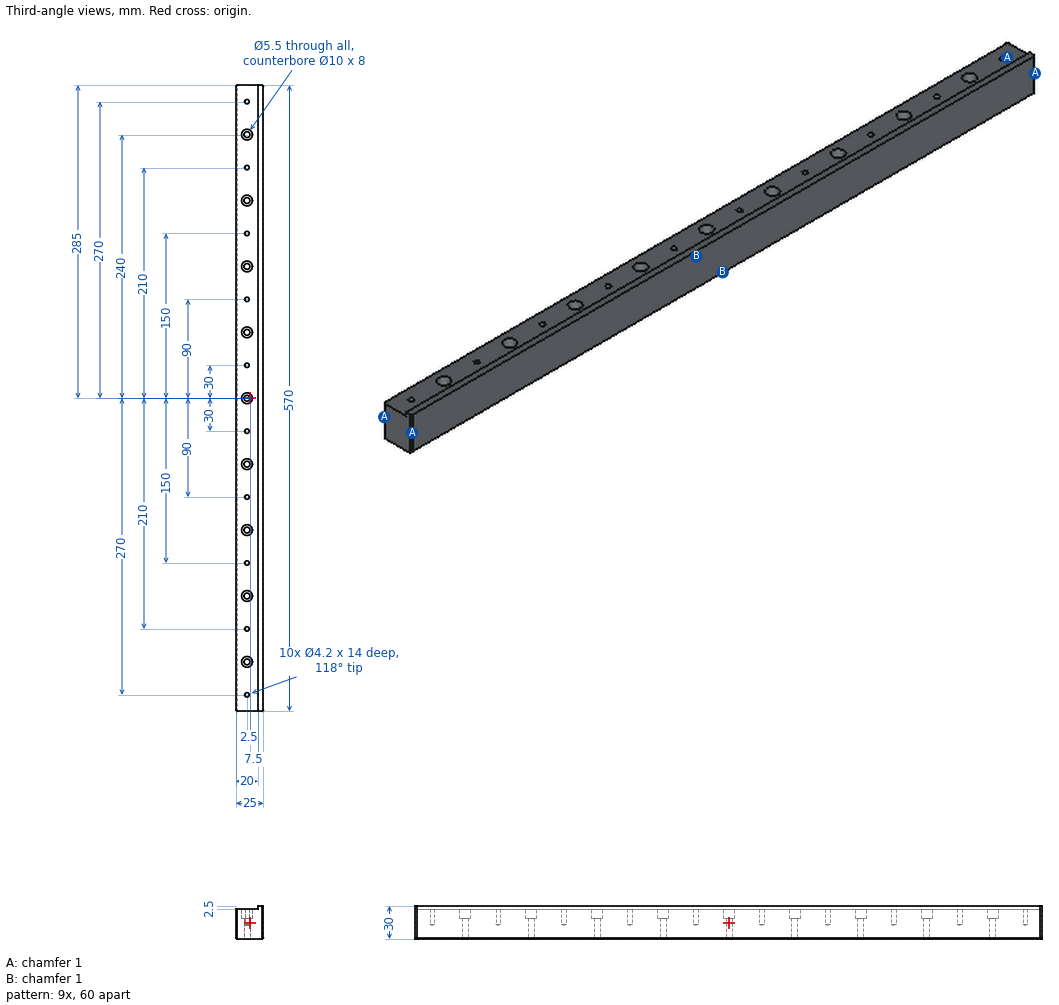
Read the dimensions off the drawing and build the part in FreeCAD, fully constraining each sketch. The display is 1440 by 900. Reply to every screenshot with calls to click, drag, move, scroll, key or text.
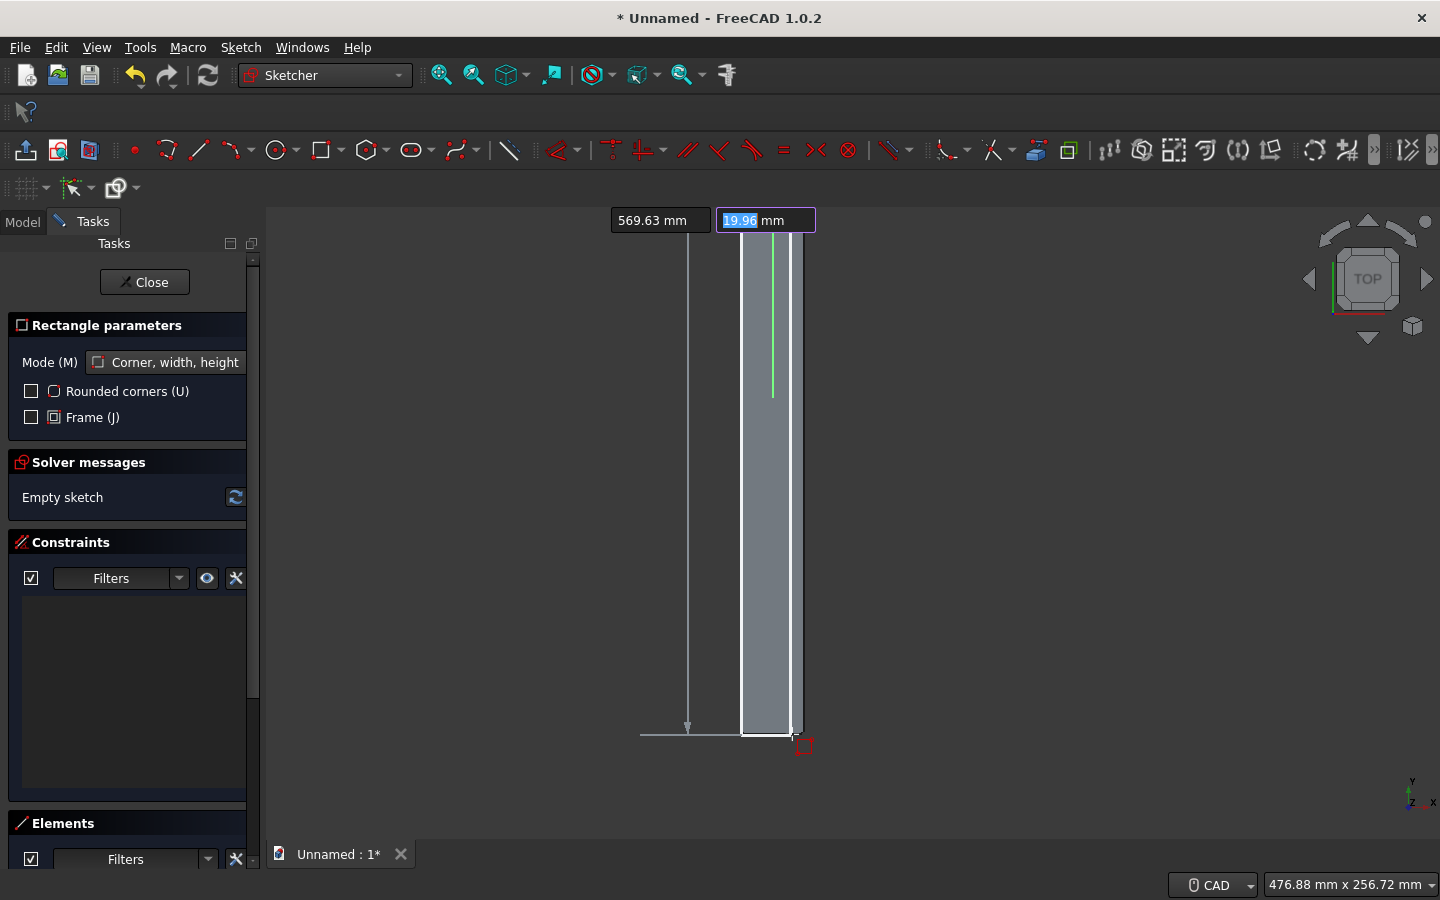
click(791, 734)
key(Escape)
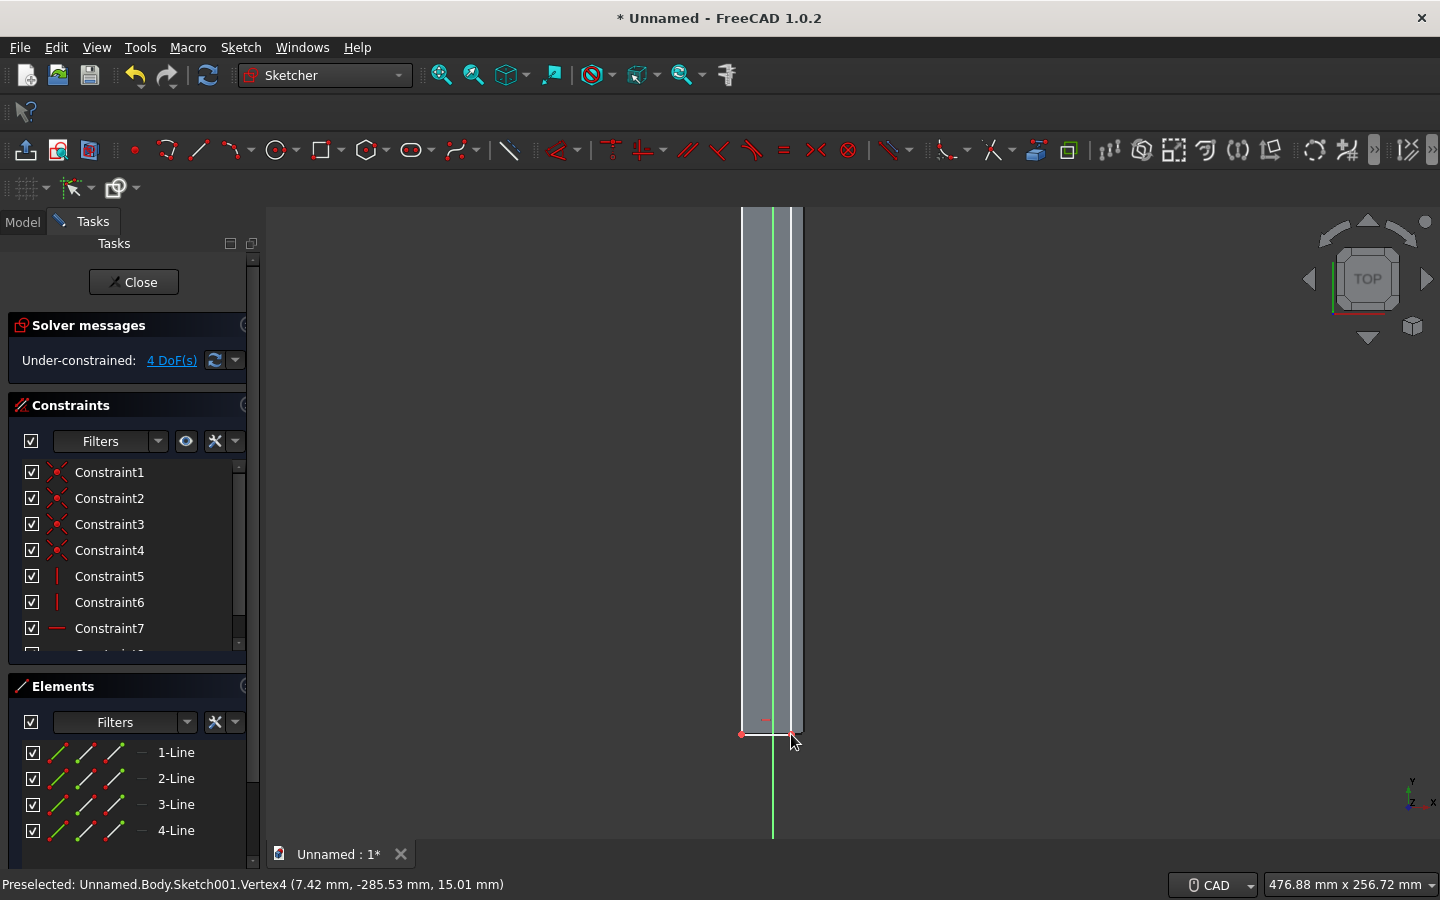
key(d)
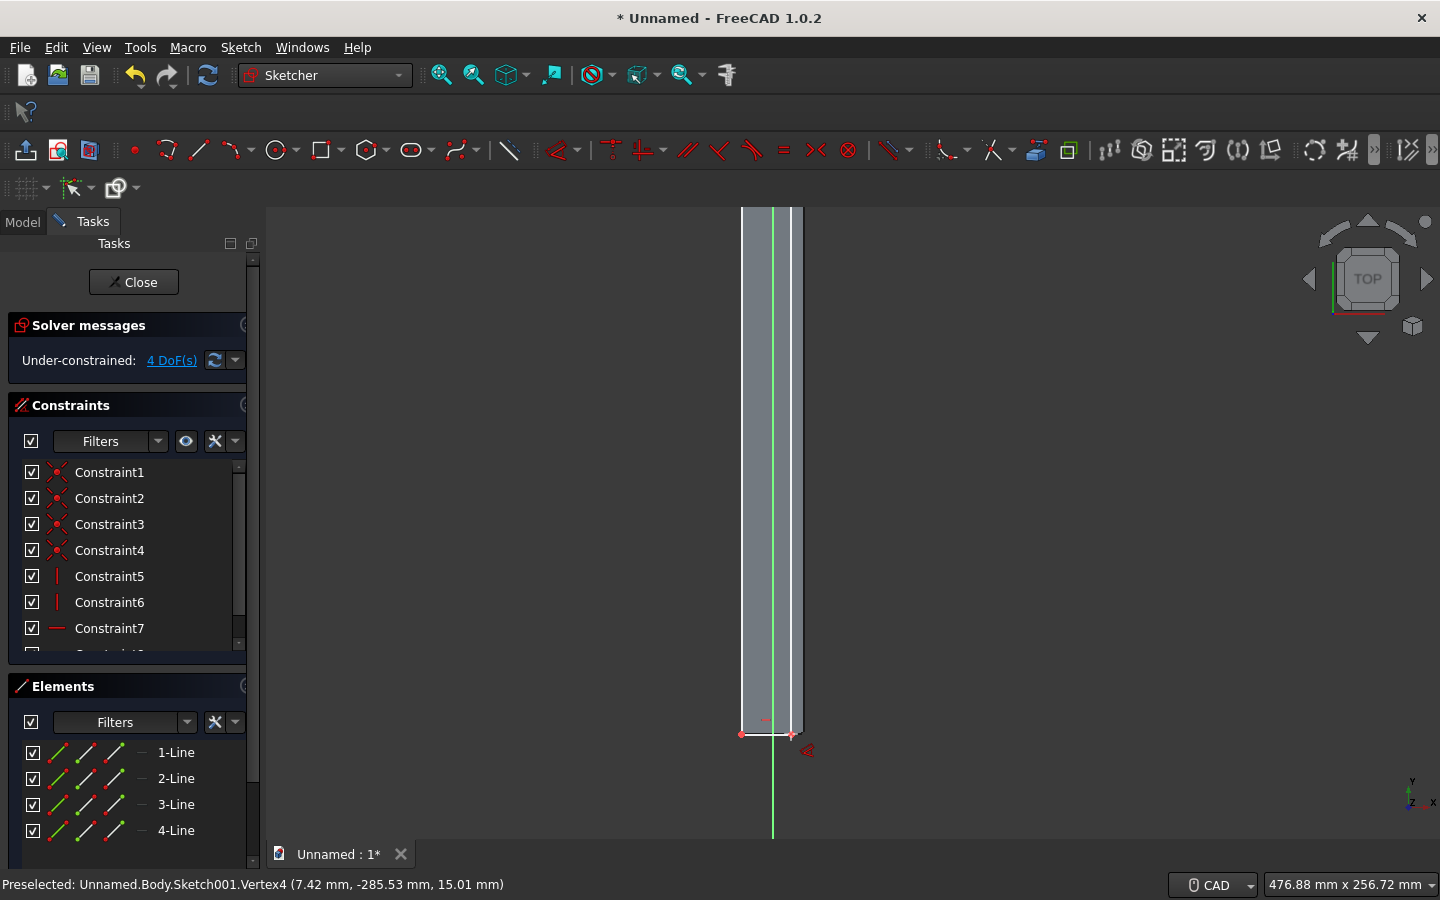
click(757, 735)
click(755, 769)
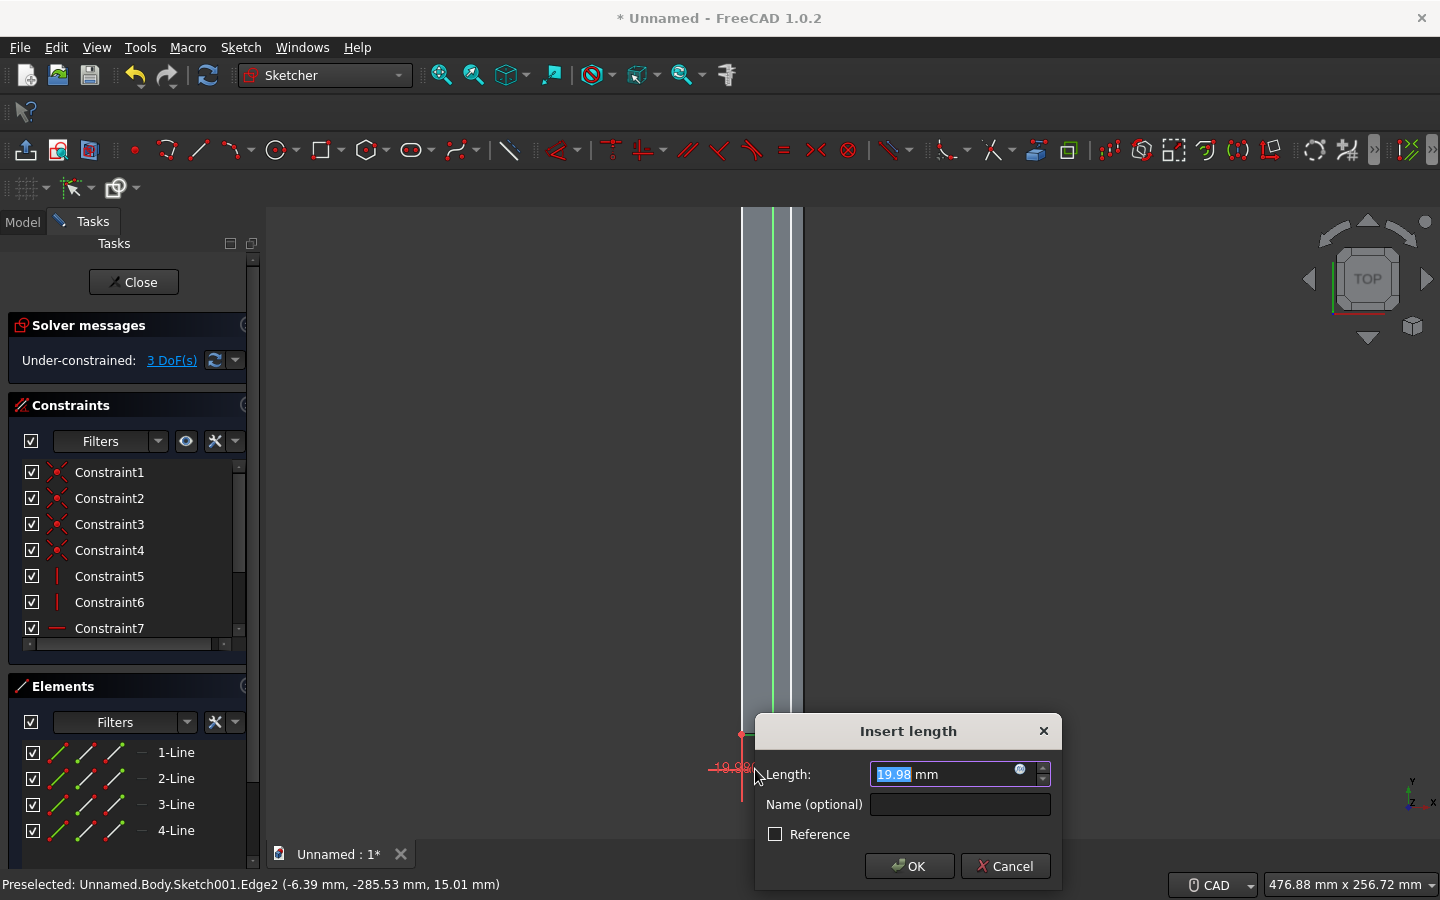
text(20)
key(Return)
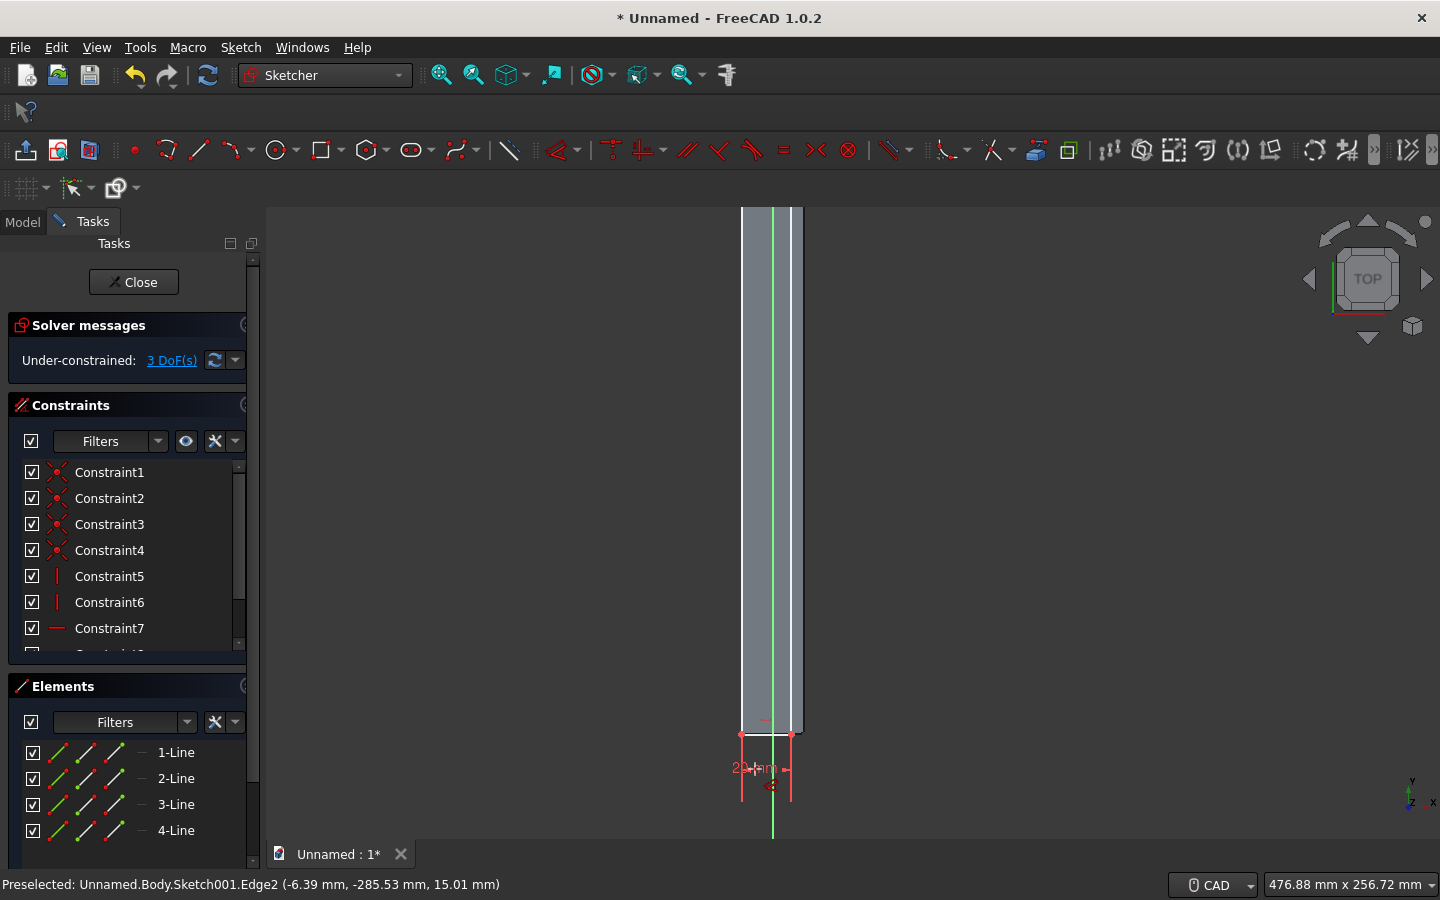
click(742, 314)
click(708, 485)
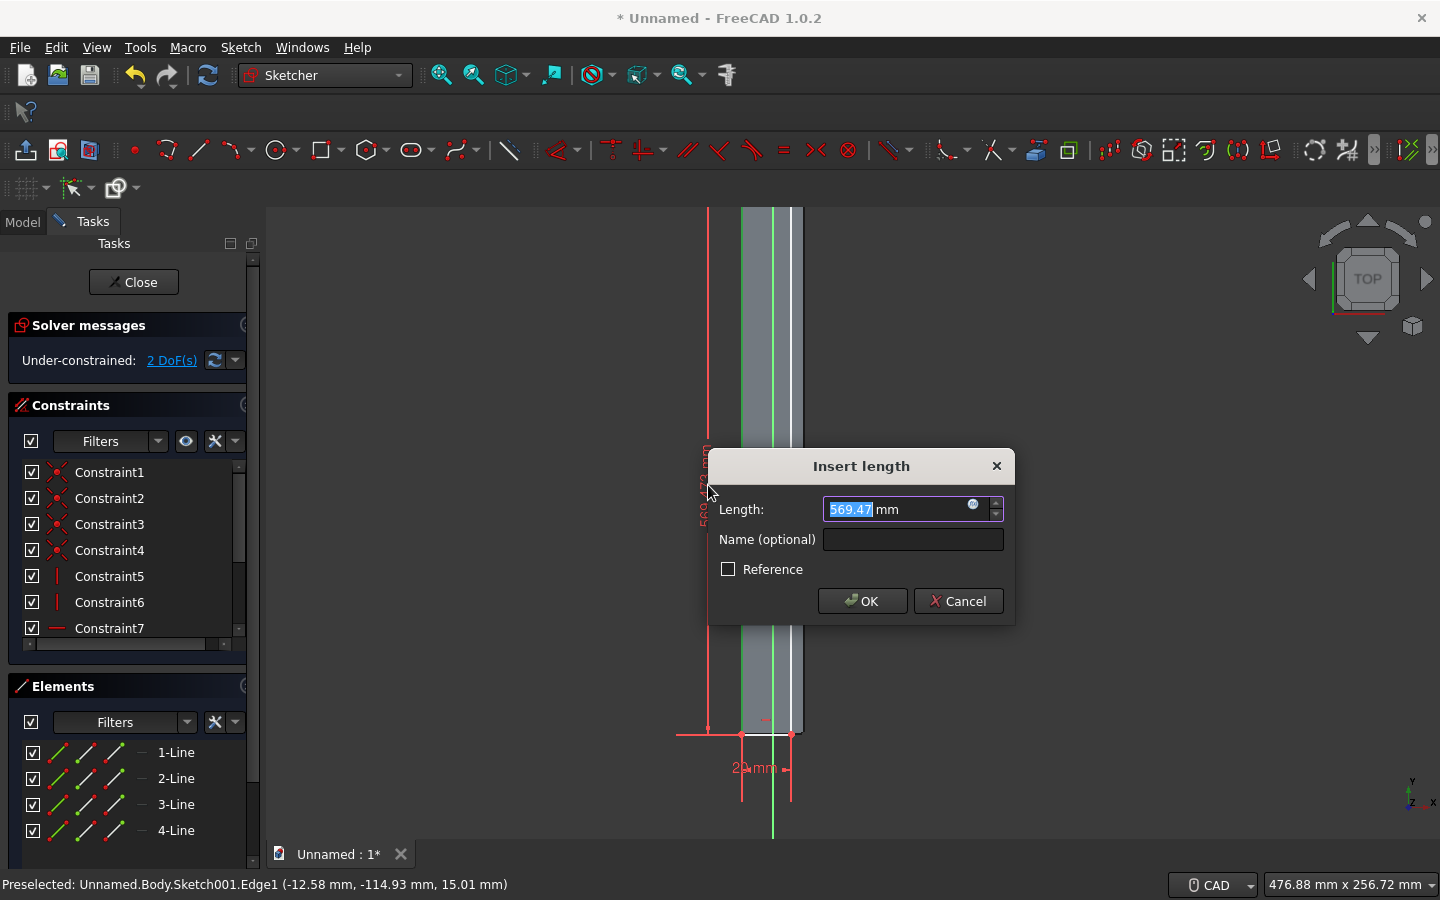
text(570)
key(Return)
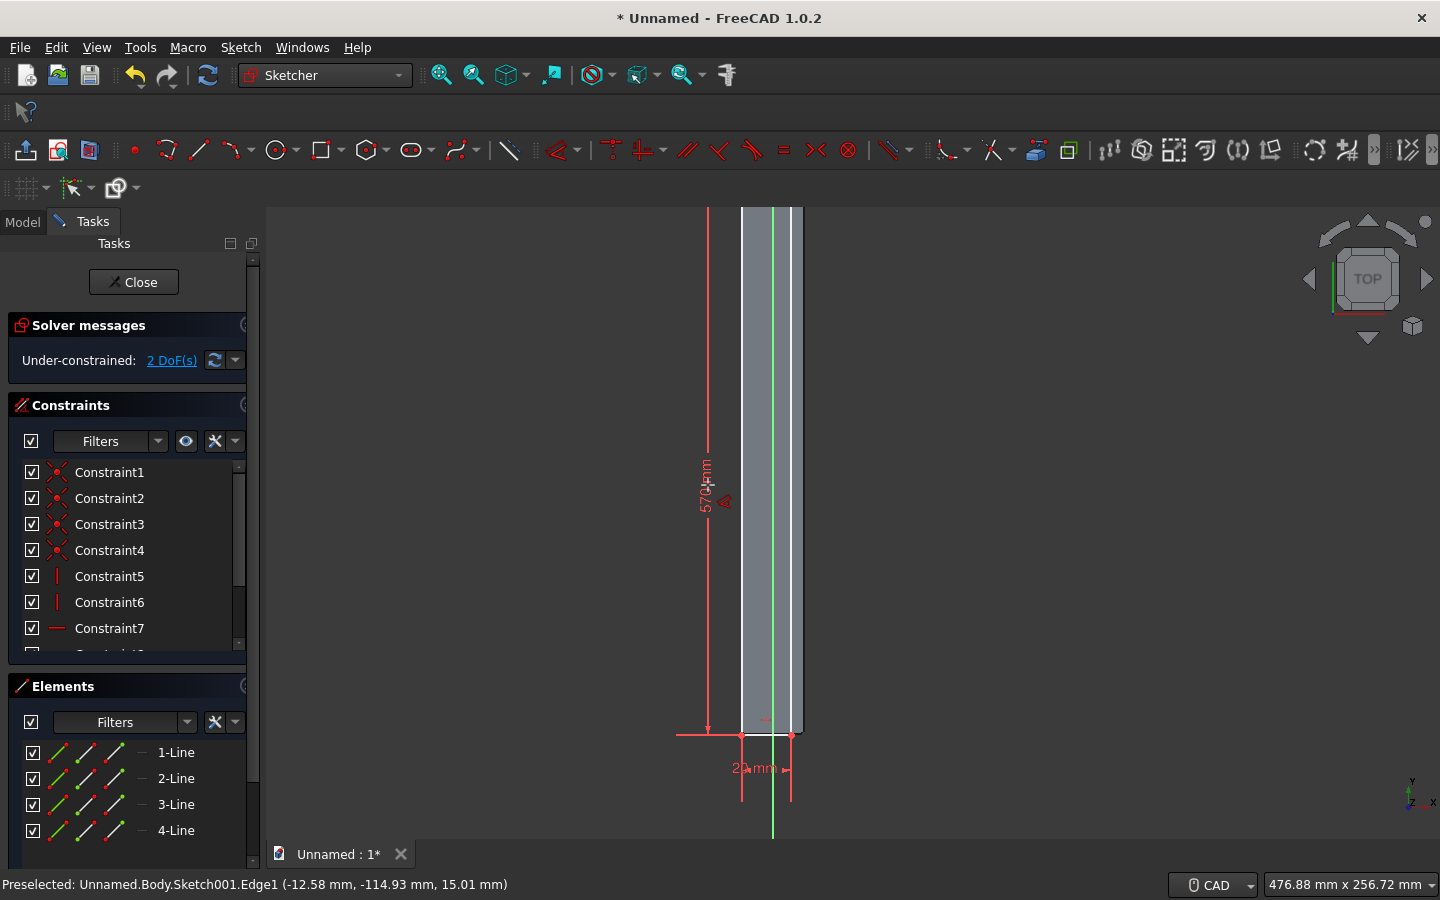
scroll(792, 735, down, 6)